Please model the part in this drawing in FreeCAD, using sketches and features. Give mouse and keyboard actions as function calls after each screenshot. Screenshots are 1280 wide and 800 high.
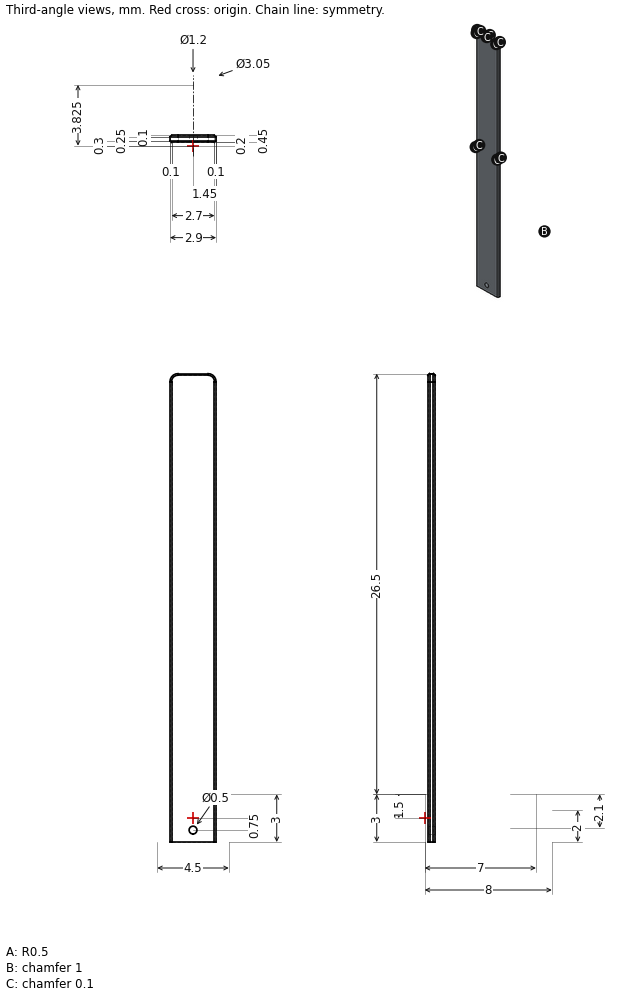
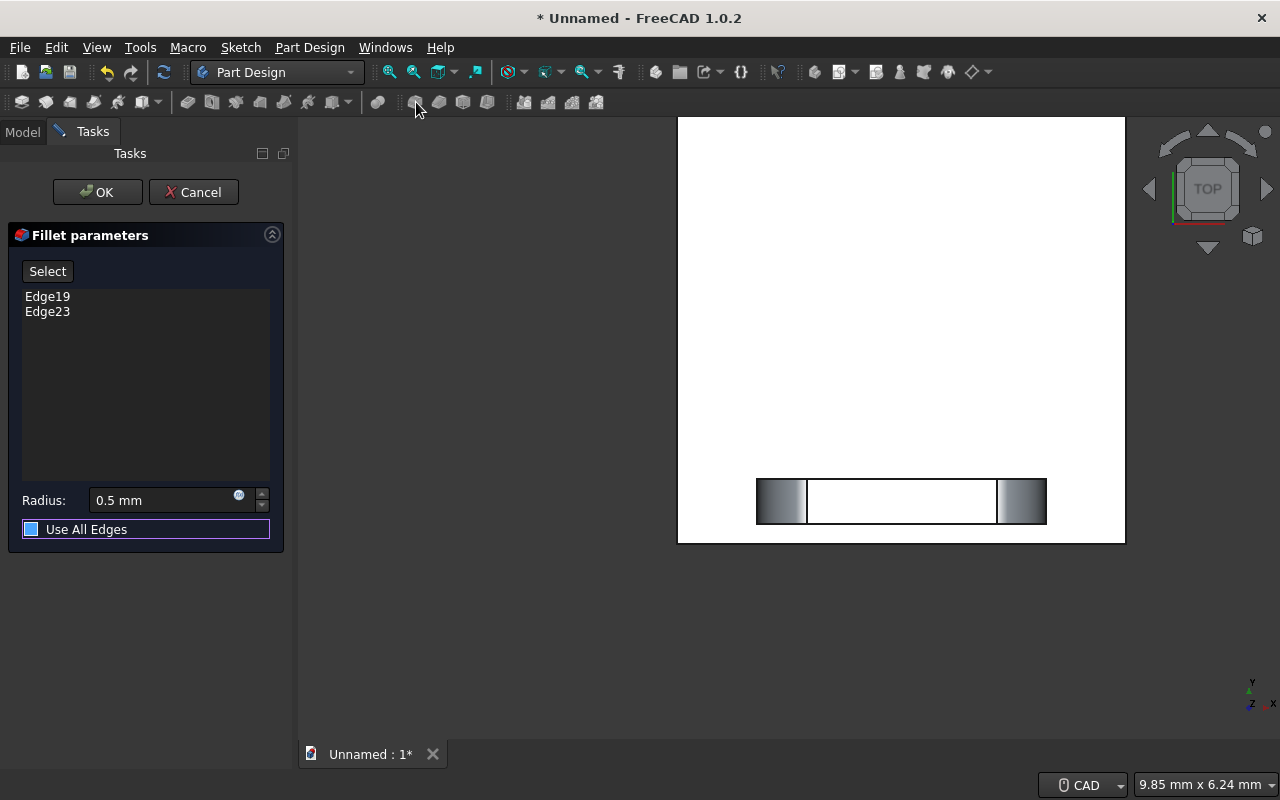
click(98, 192)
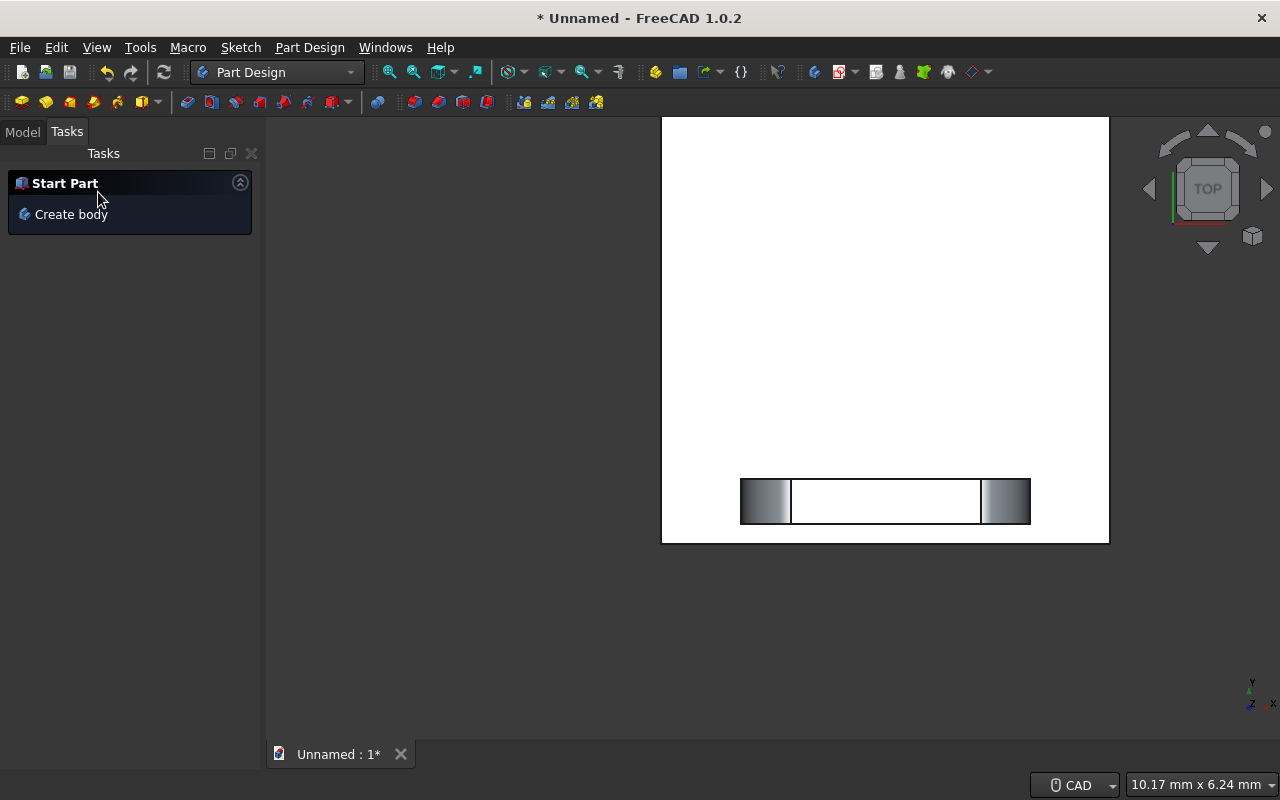
key(v)
key(f)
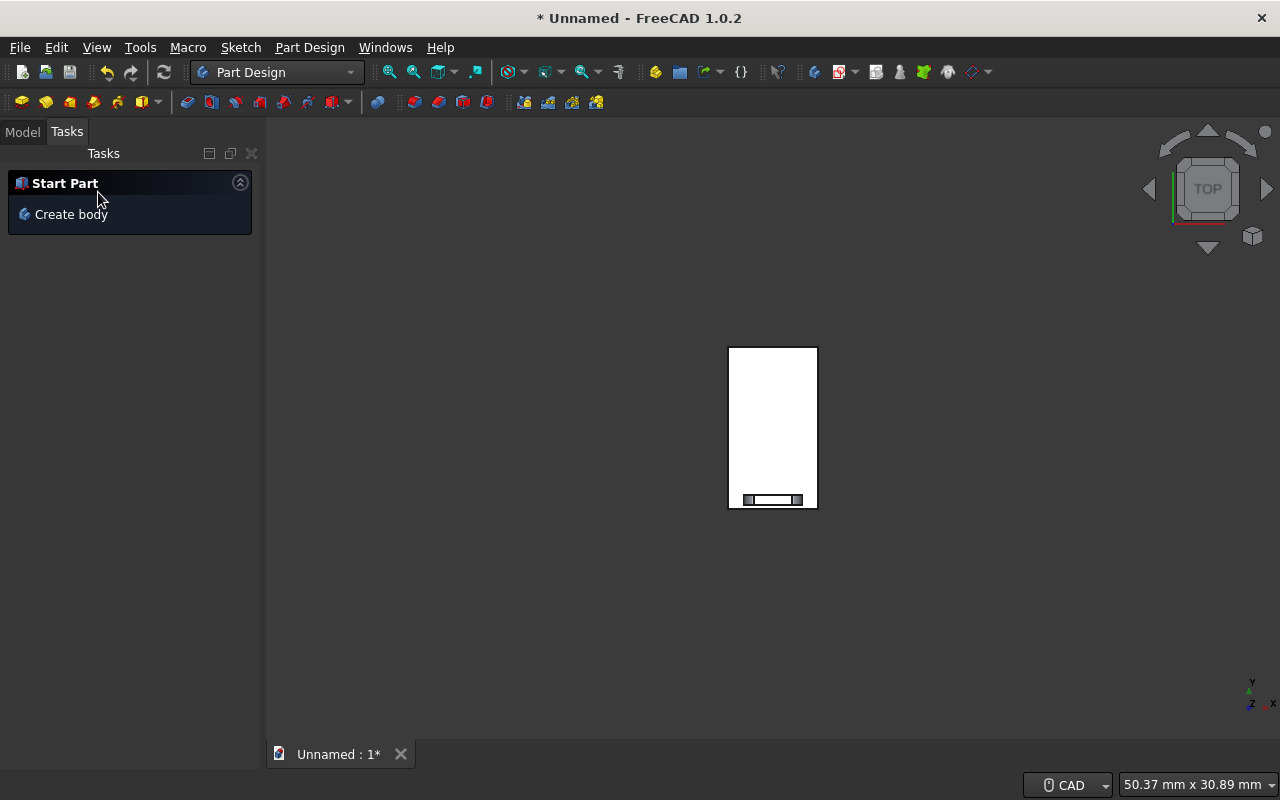
click(773, 346)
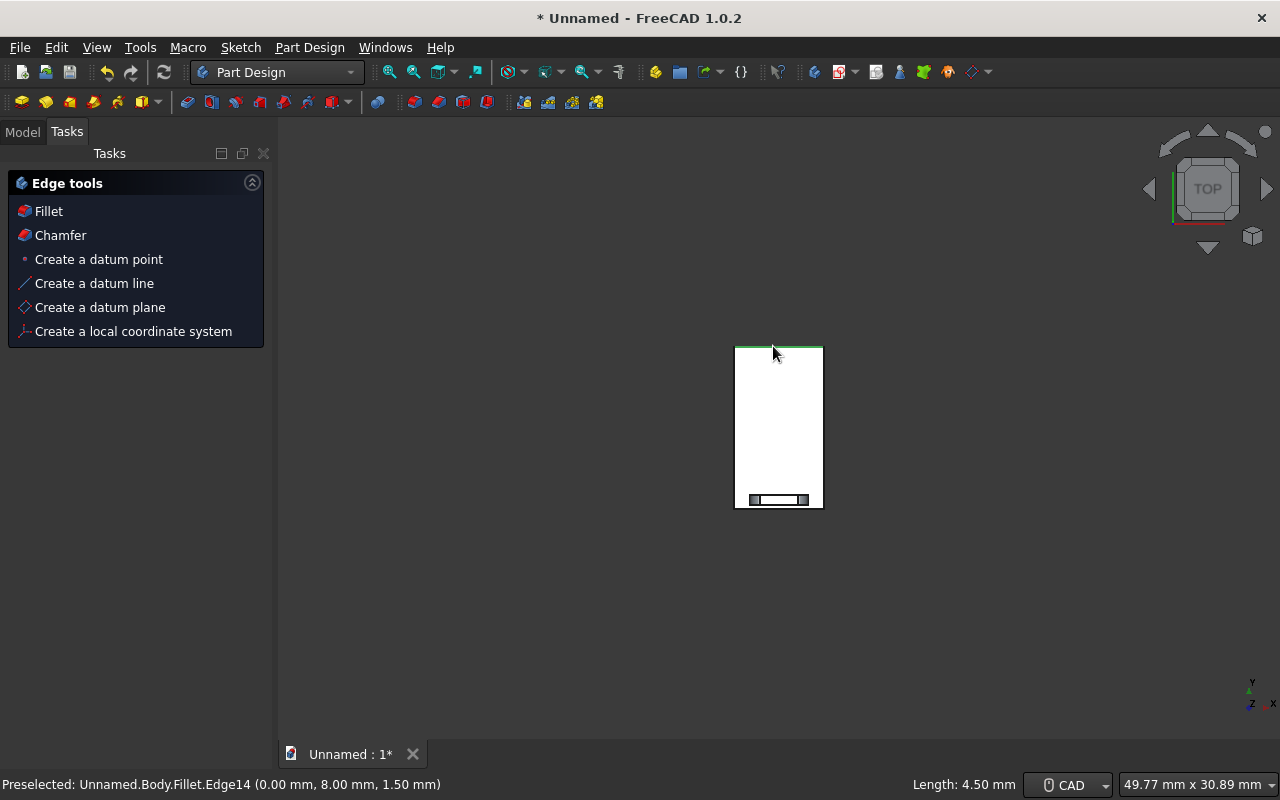
click(440, 102)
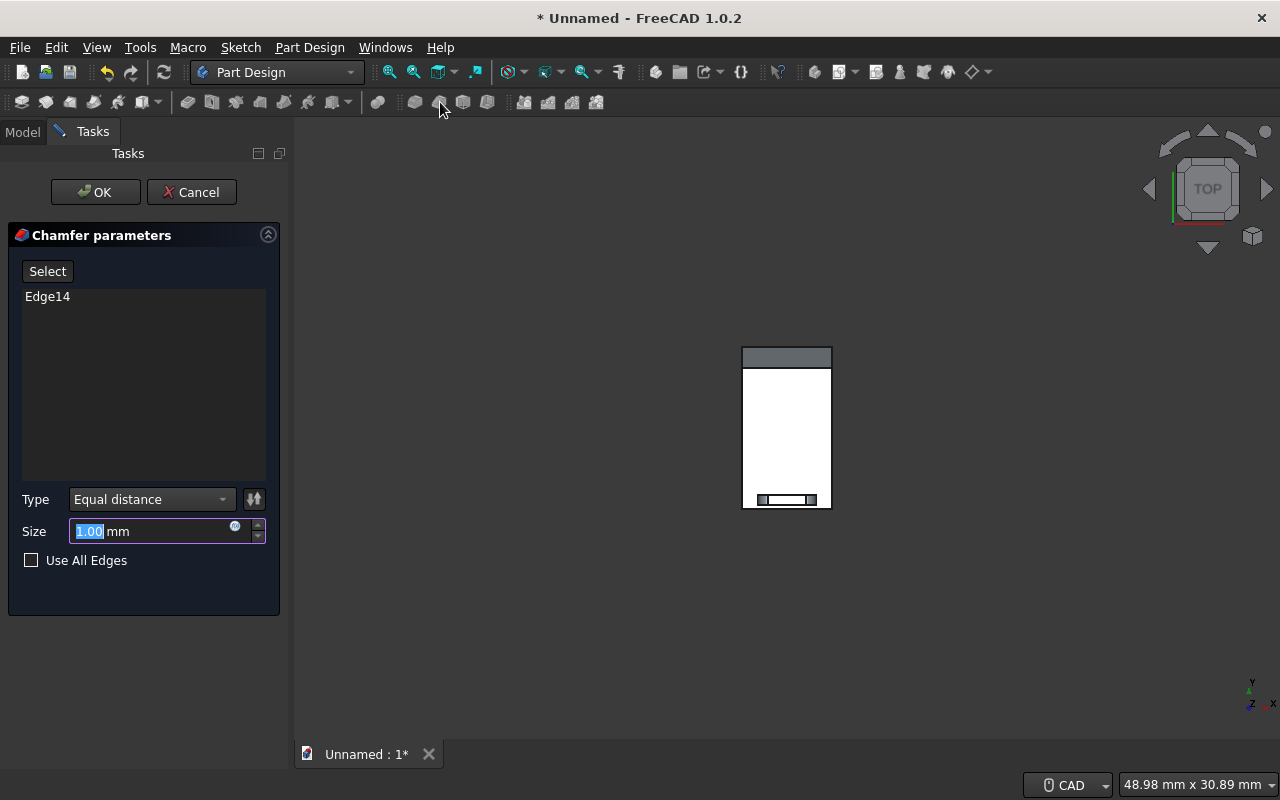
text(1)
key(Tab)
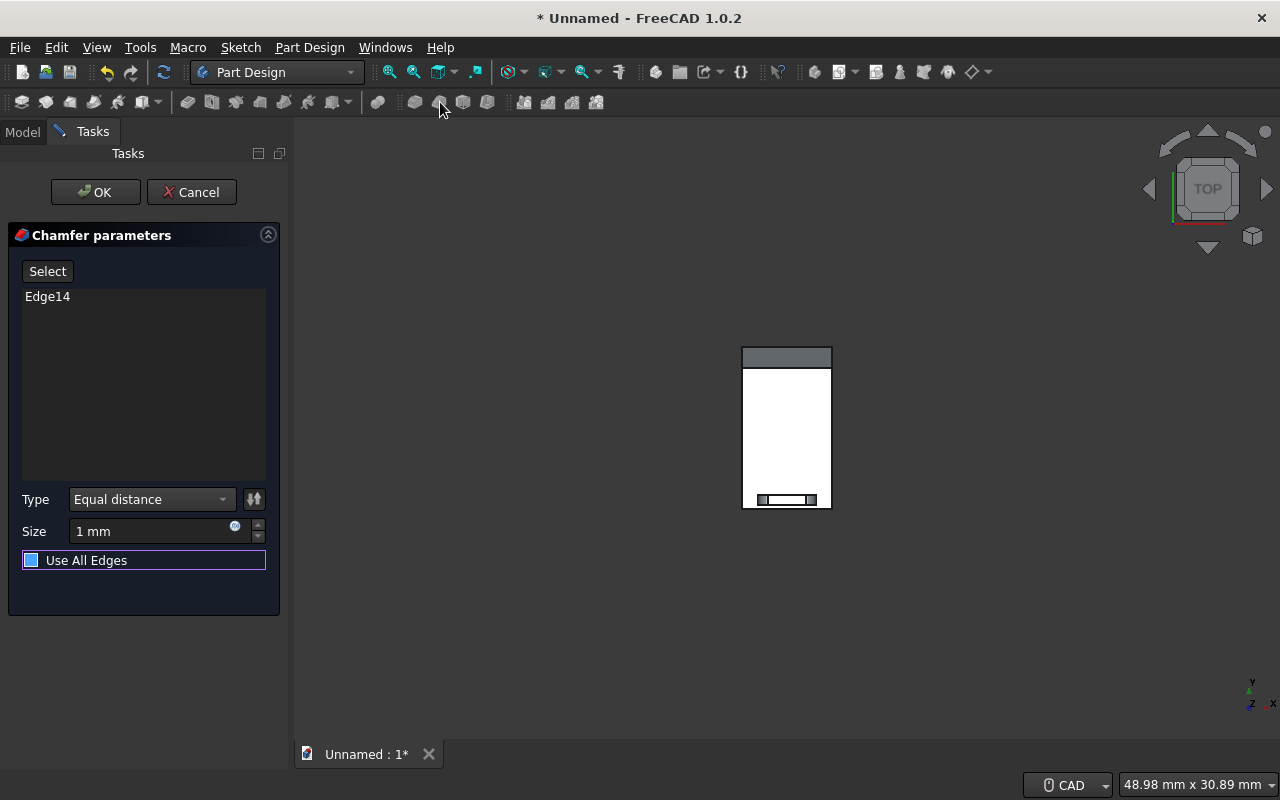
click(96, 192)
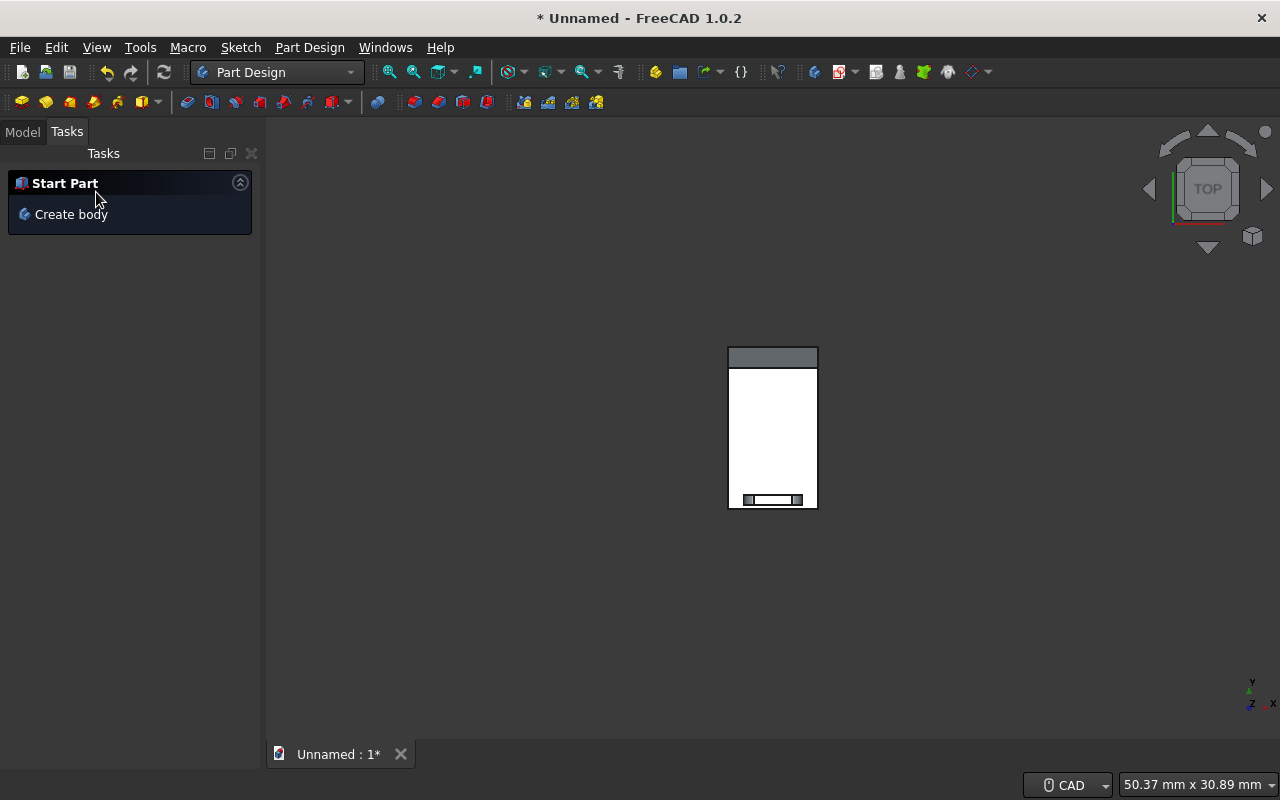
key(v)
key(f)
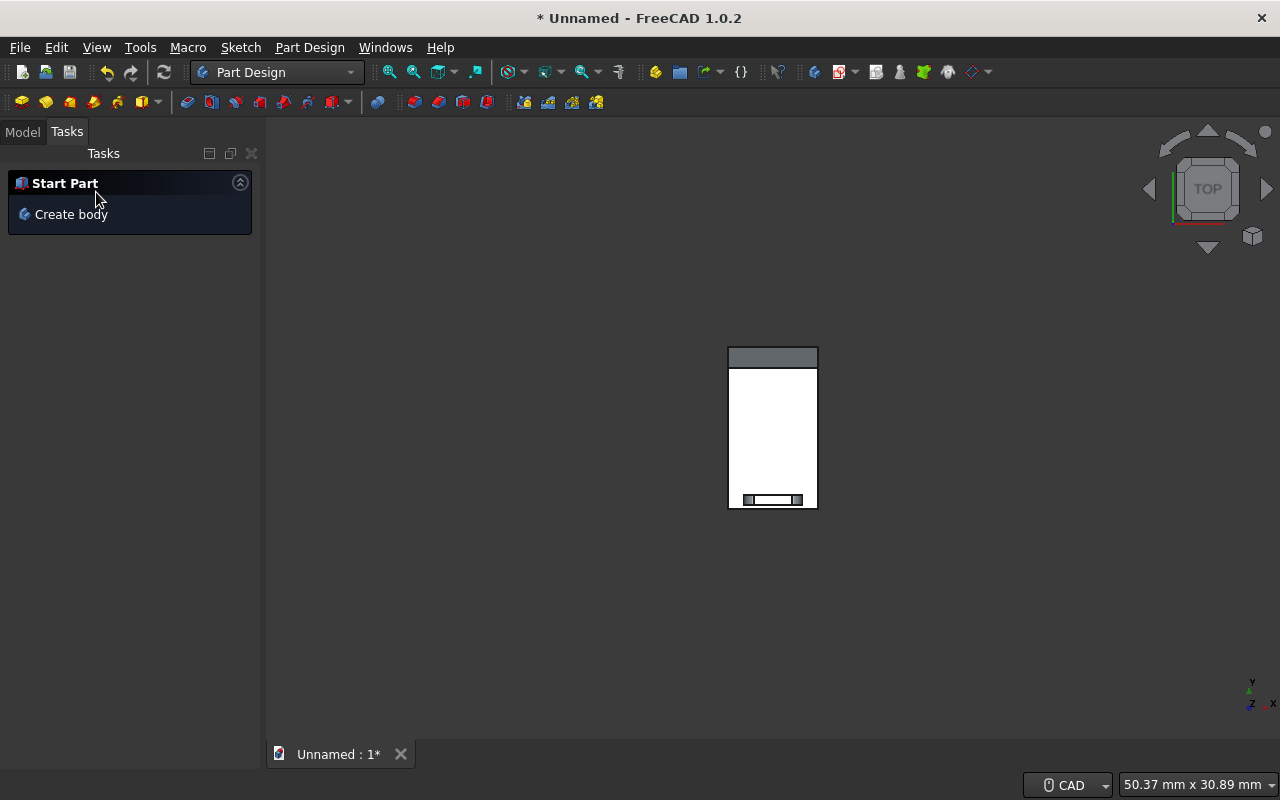
click(773, 494)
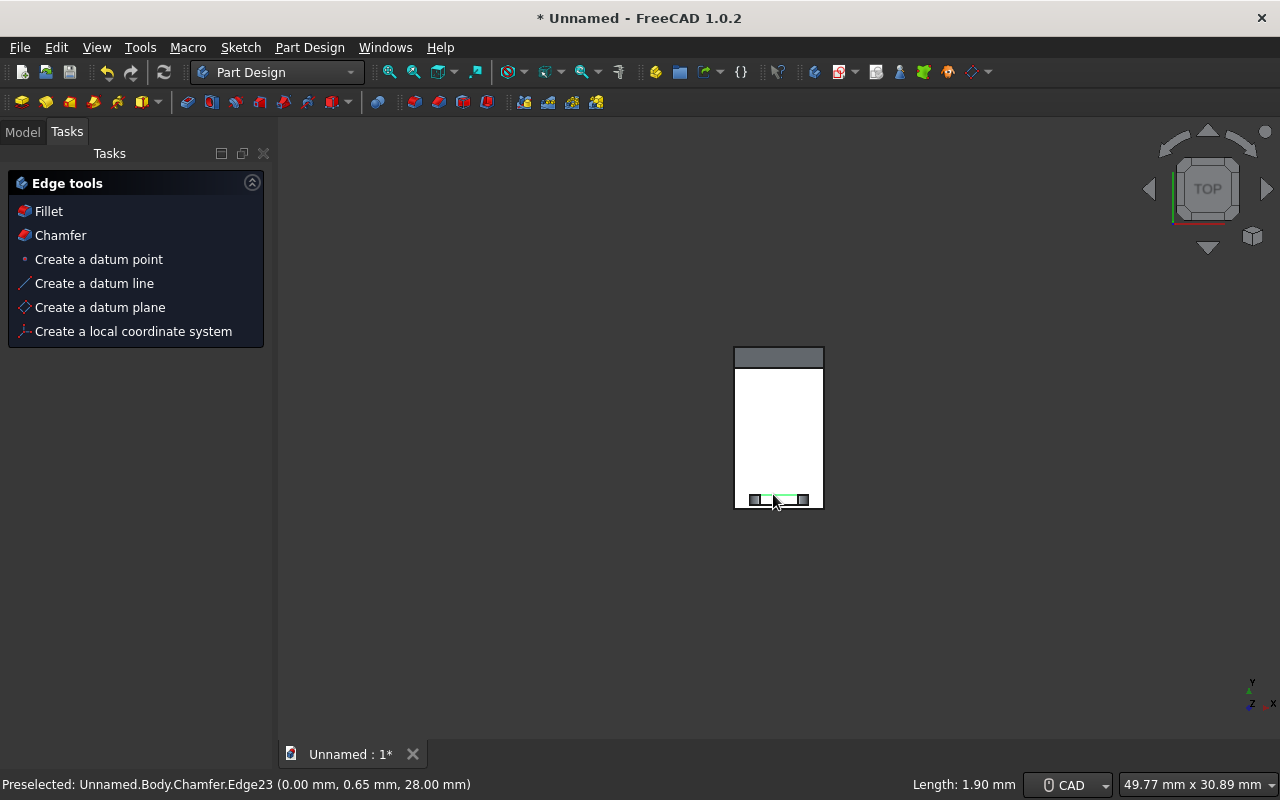
click(805, 504, ctrl)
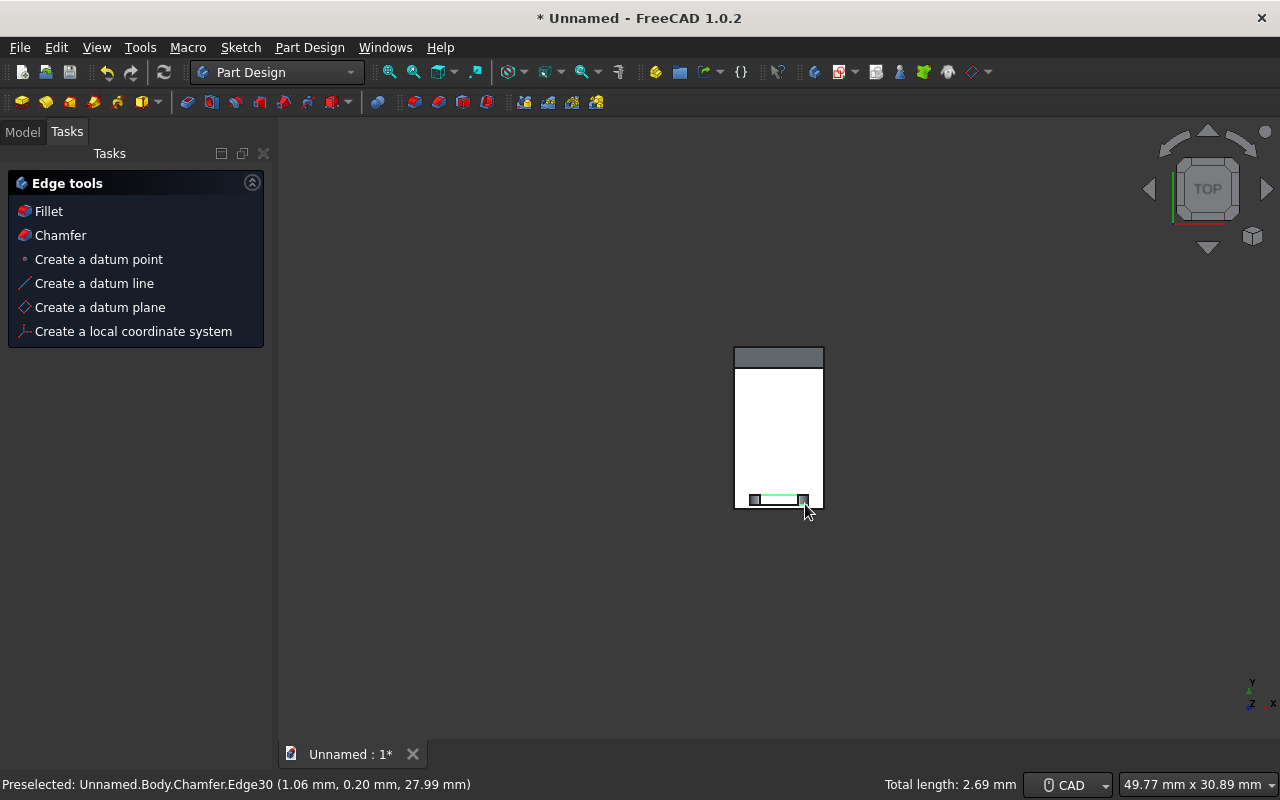
click(753, 504, ctrl)